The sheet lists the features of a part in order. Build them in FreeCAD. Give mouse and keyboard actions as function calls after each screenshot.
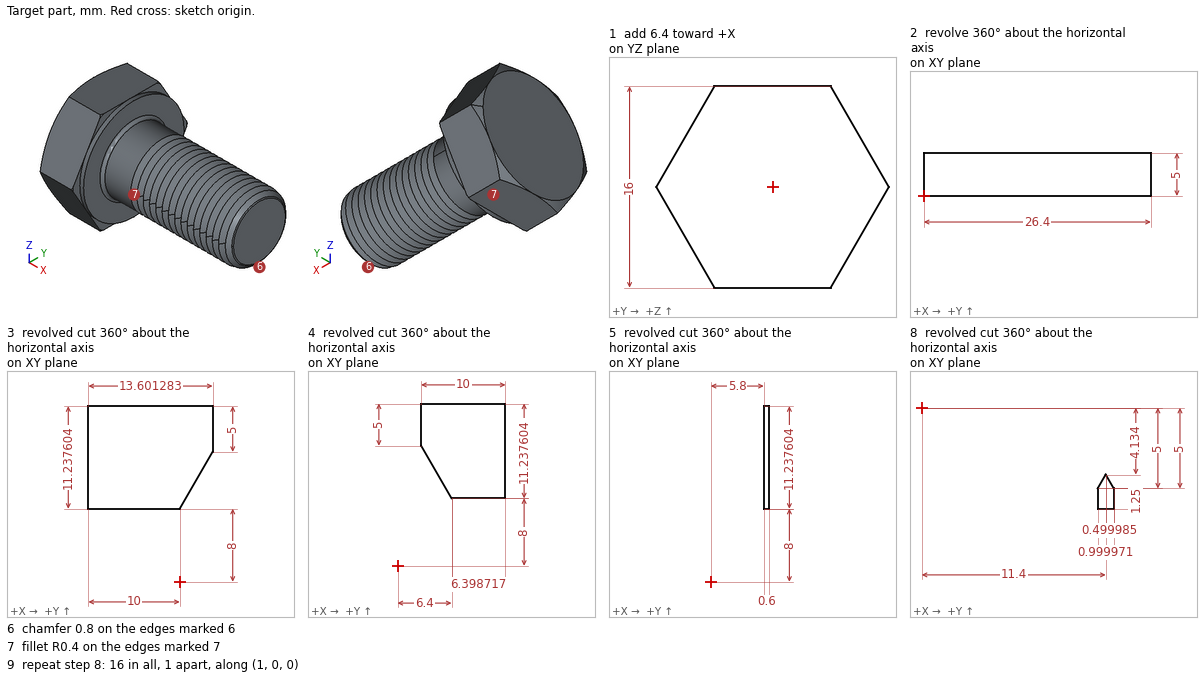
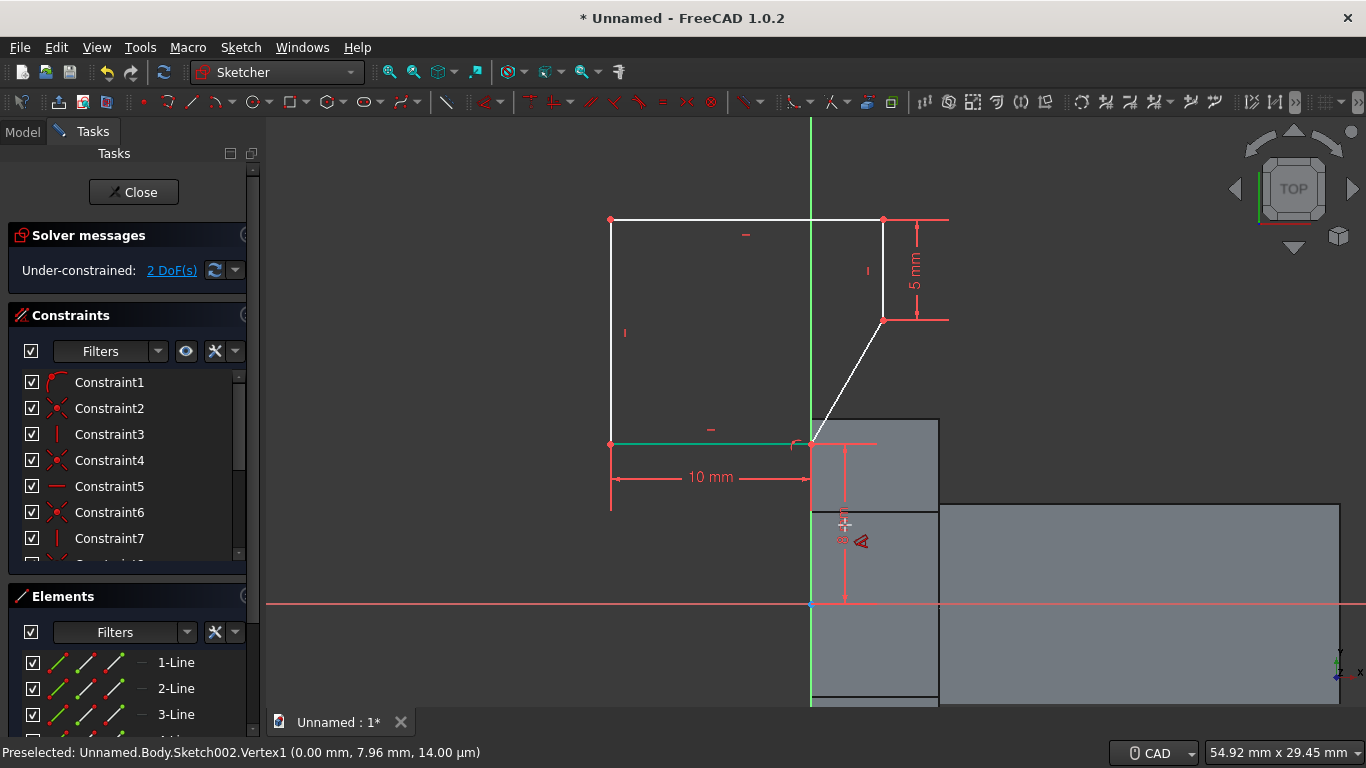
scroll(801, 220, up, 2)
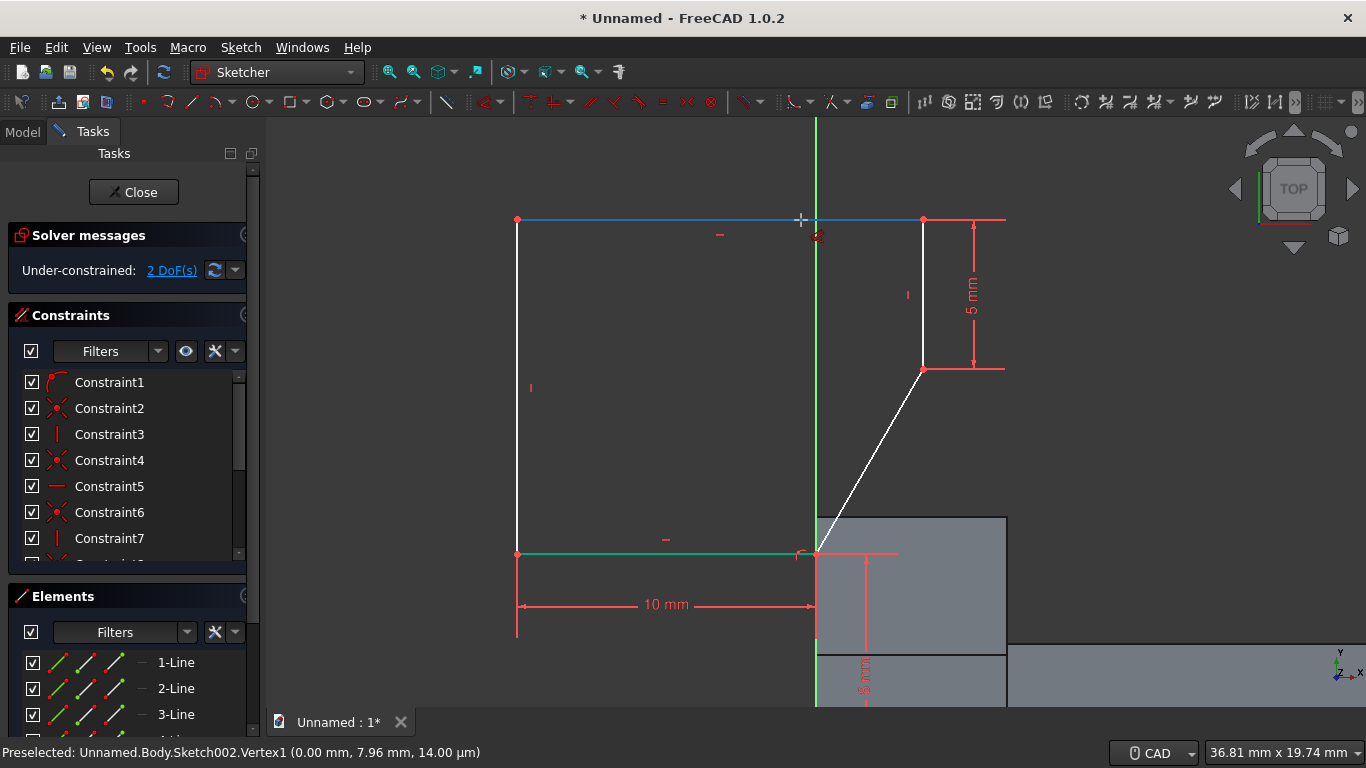
click(801, 220)
click(720, 186)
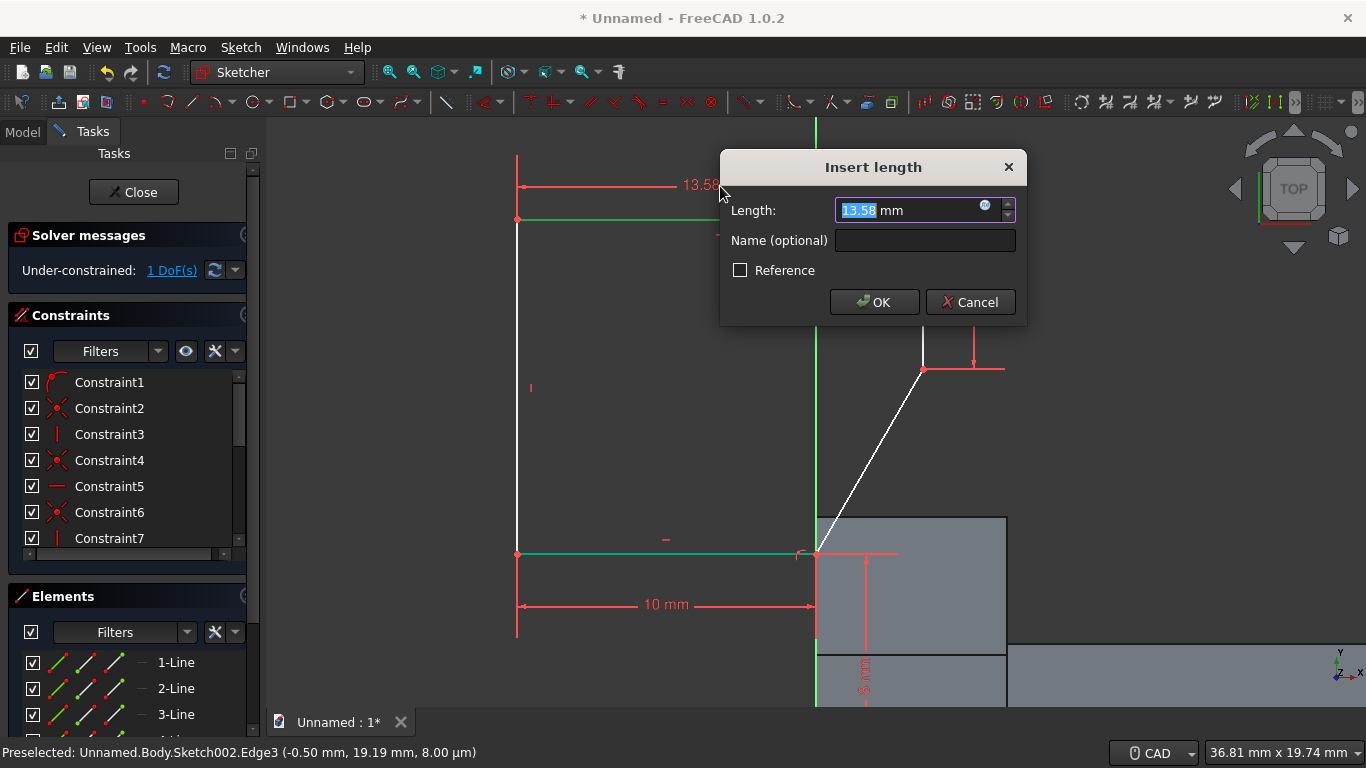
text(13.601283)
key(Return)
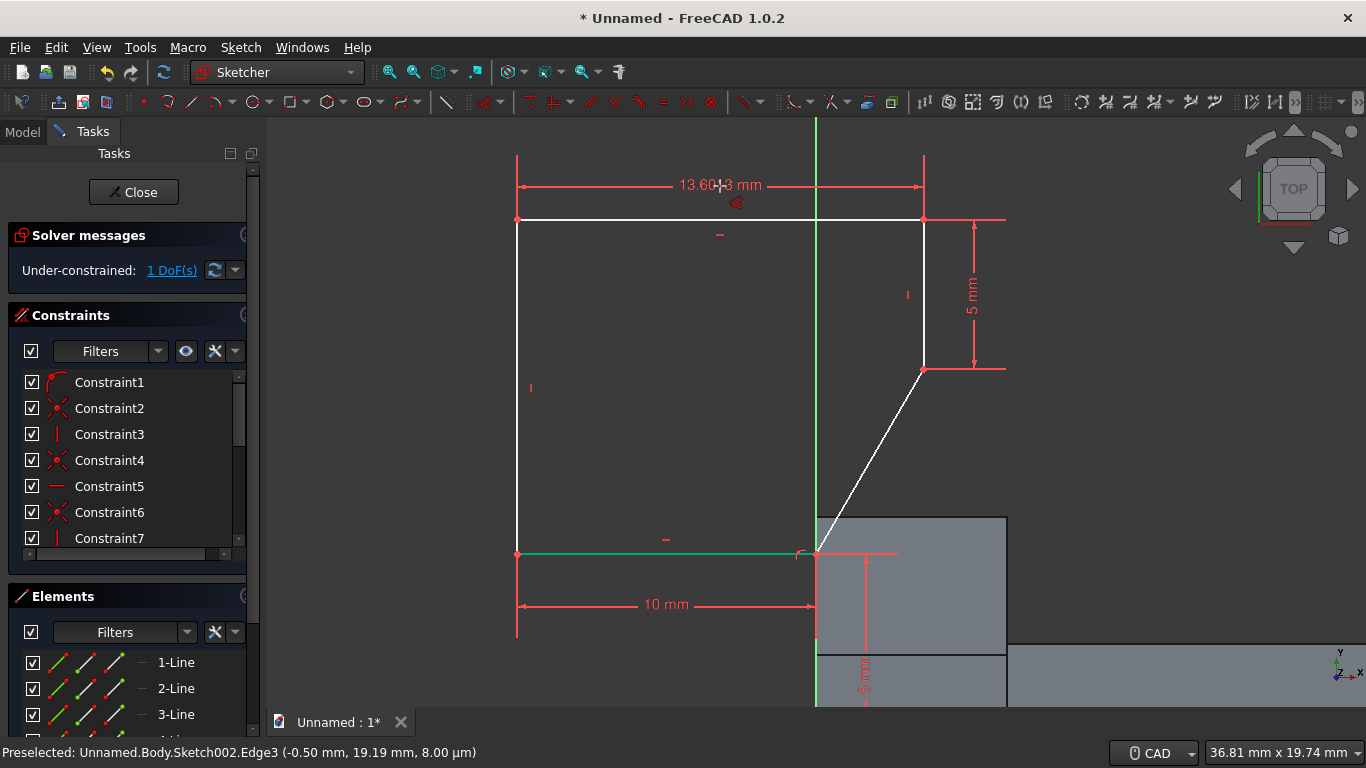
click(517, 320)
click(483, 387)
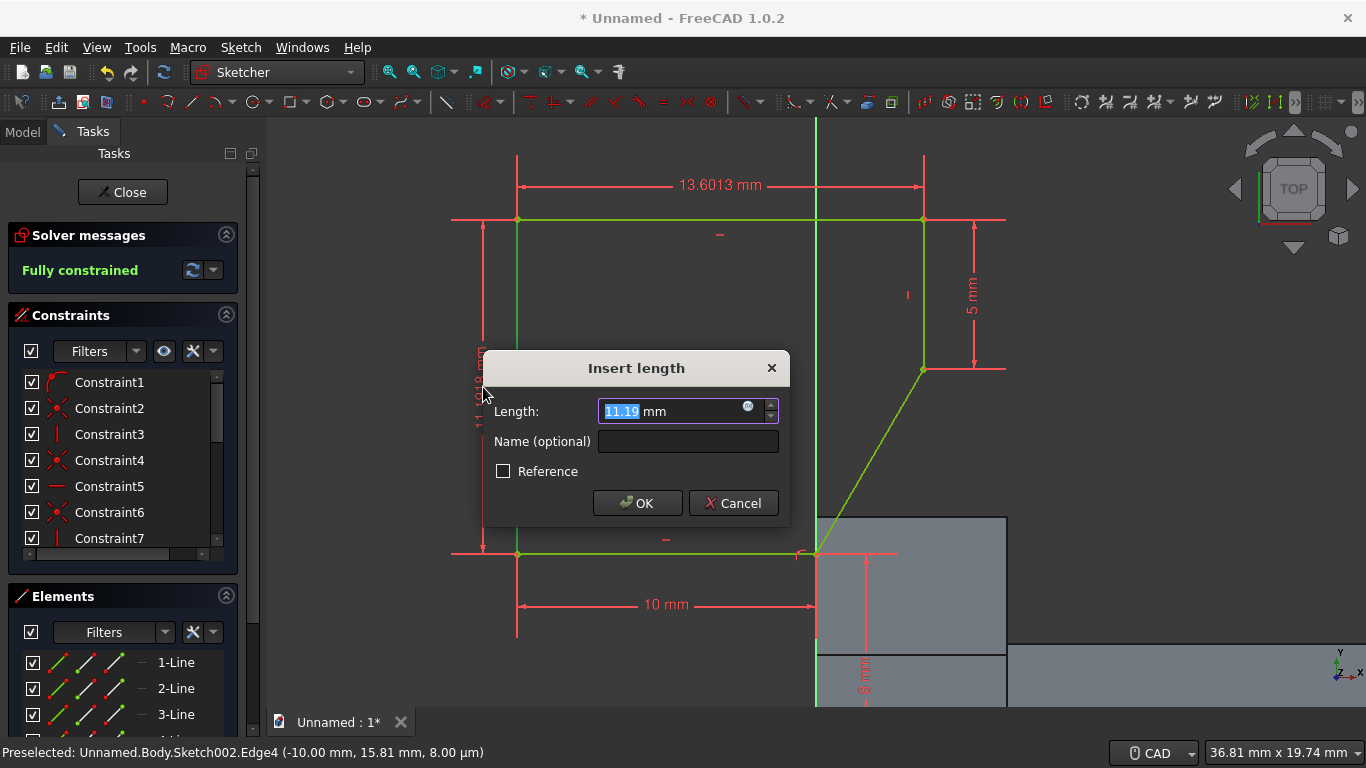
text(11.237604)
key(Return)
key(Escape)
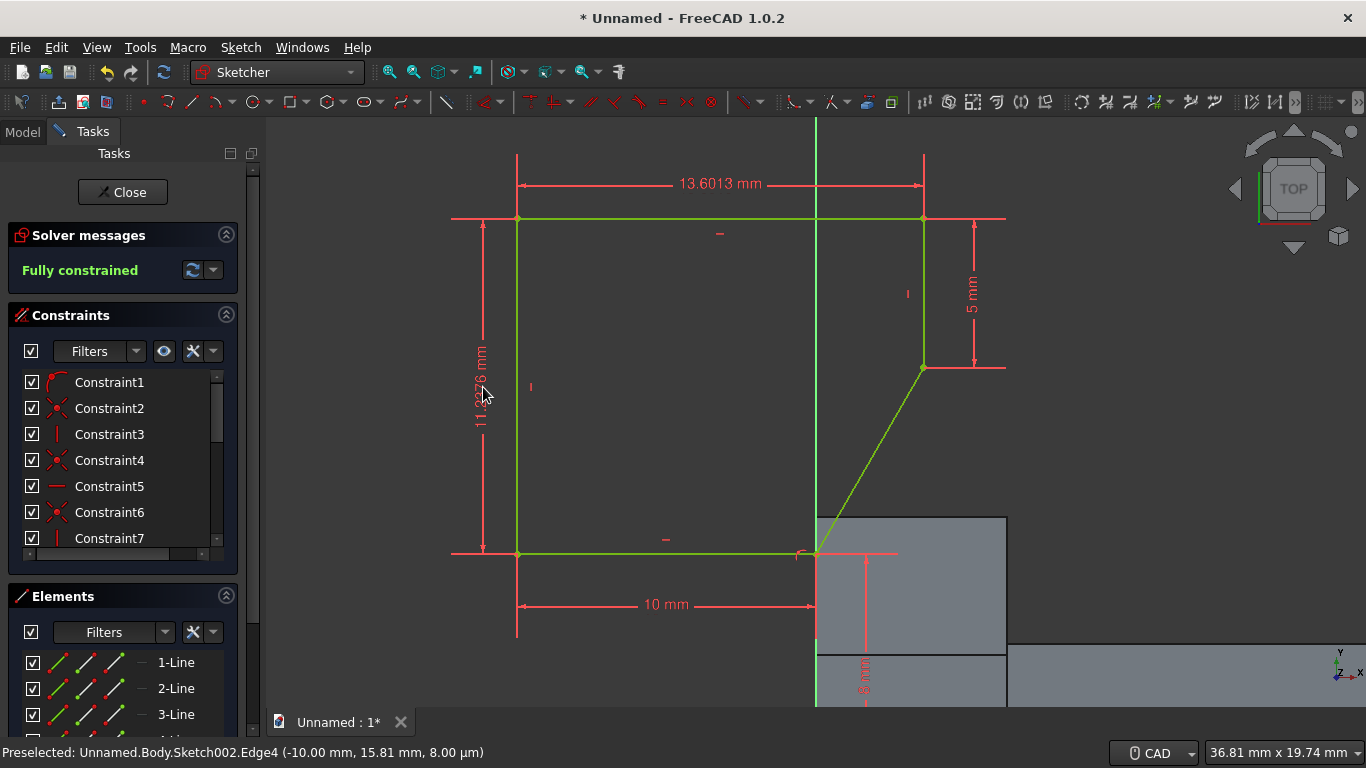
click(123, 192)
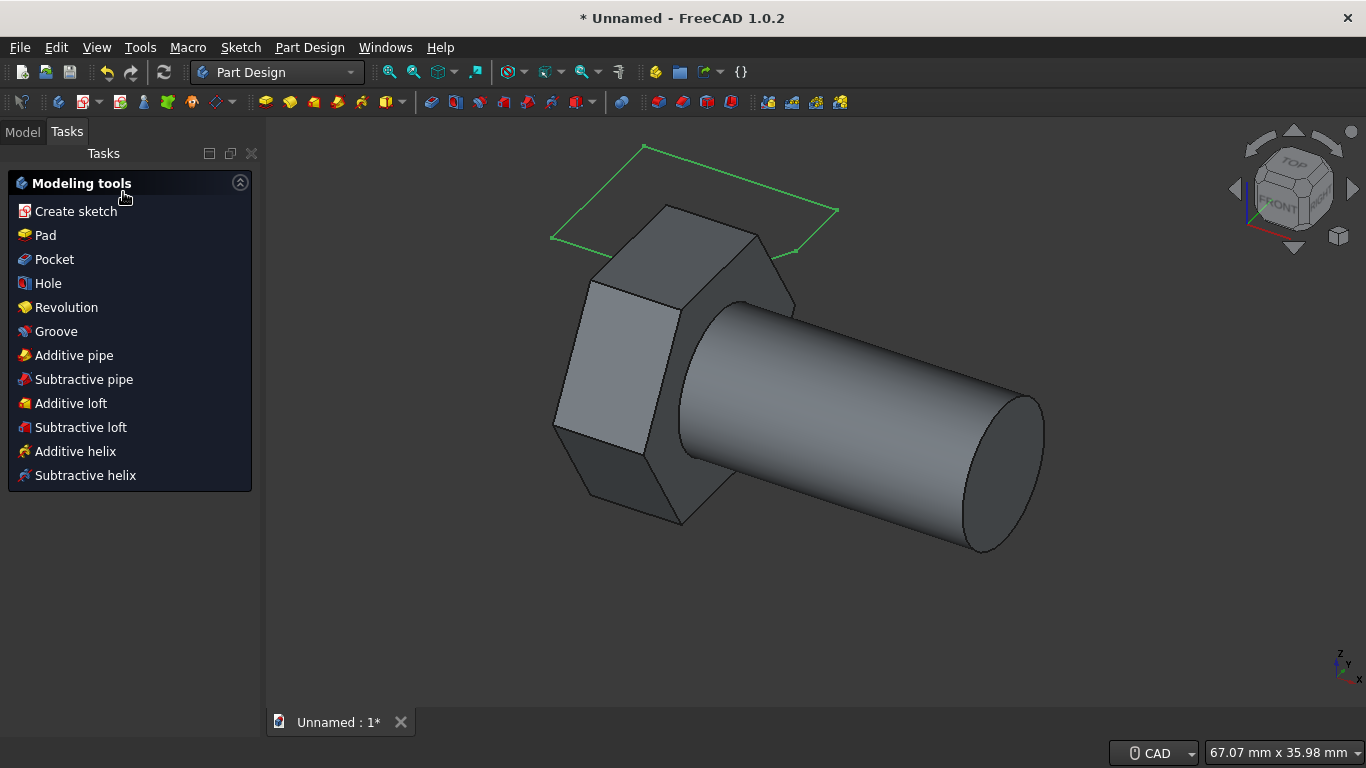
click(480, 102)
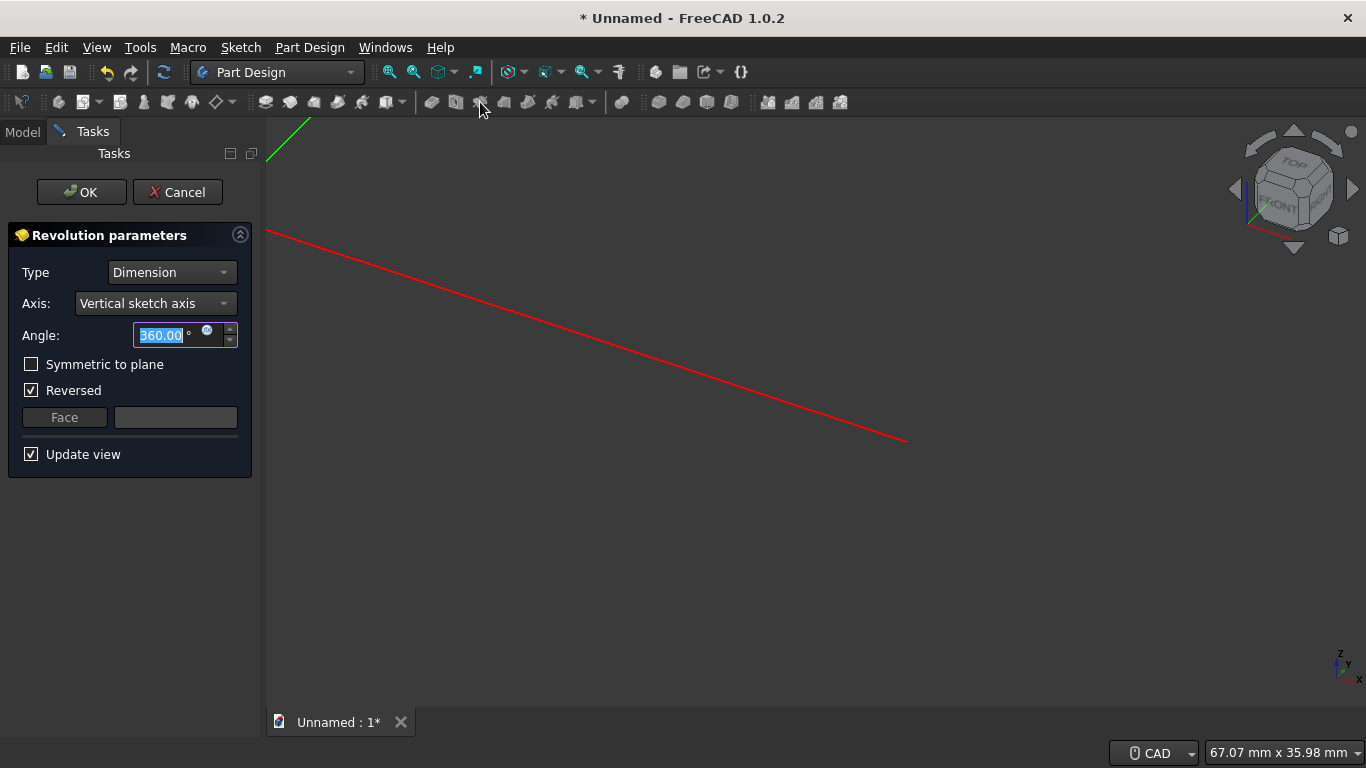
click(156, 304)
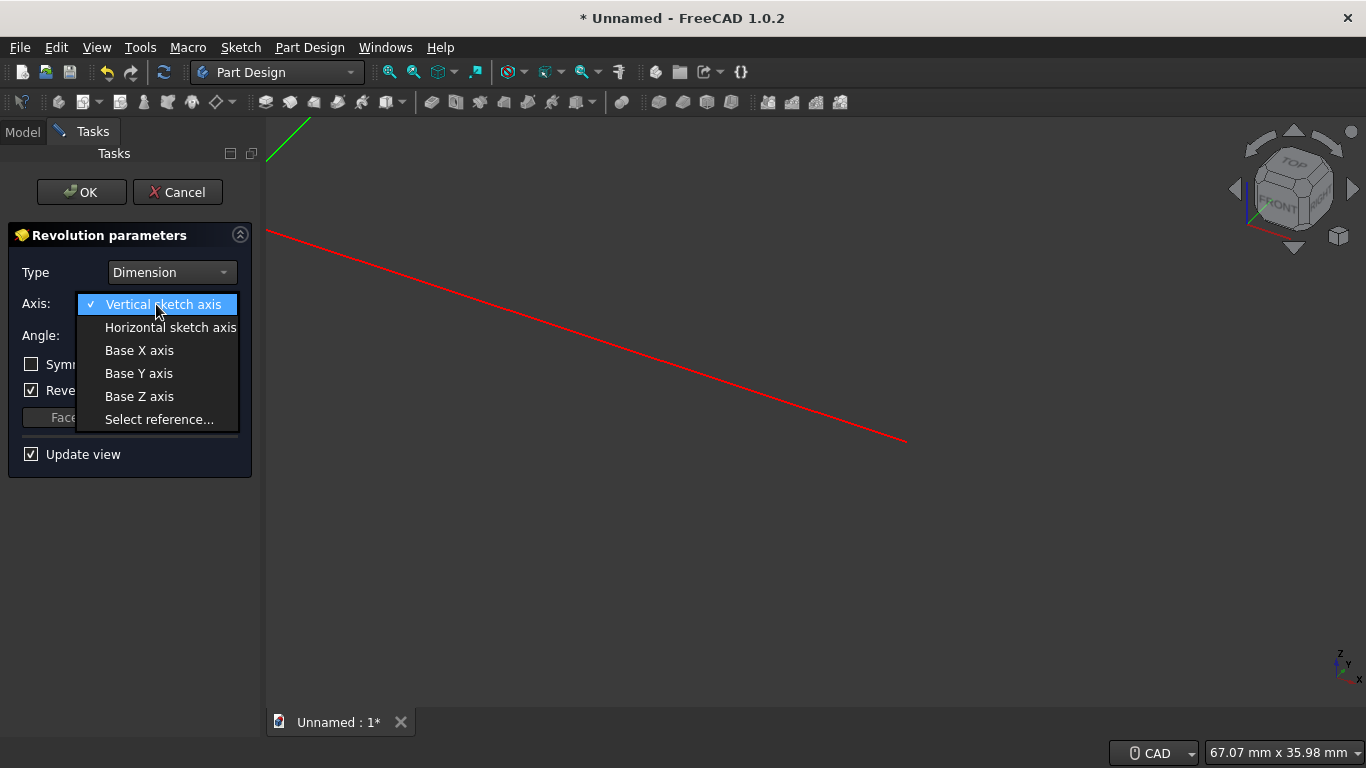
click(156, 328)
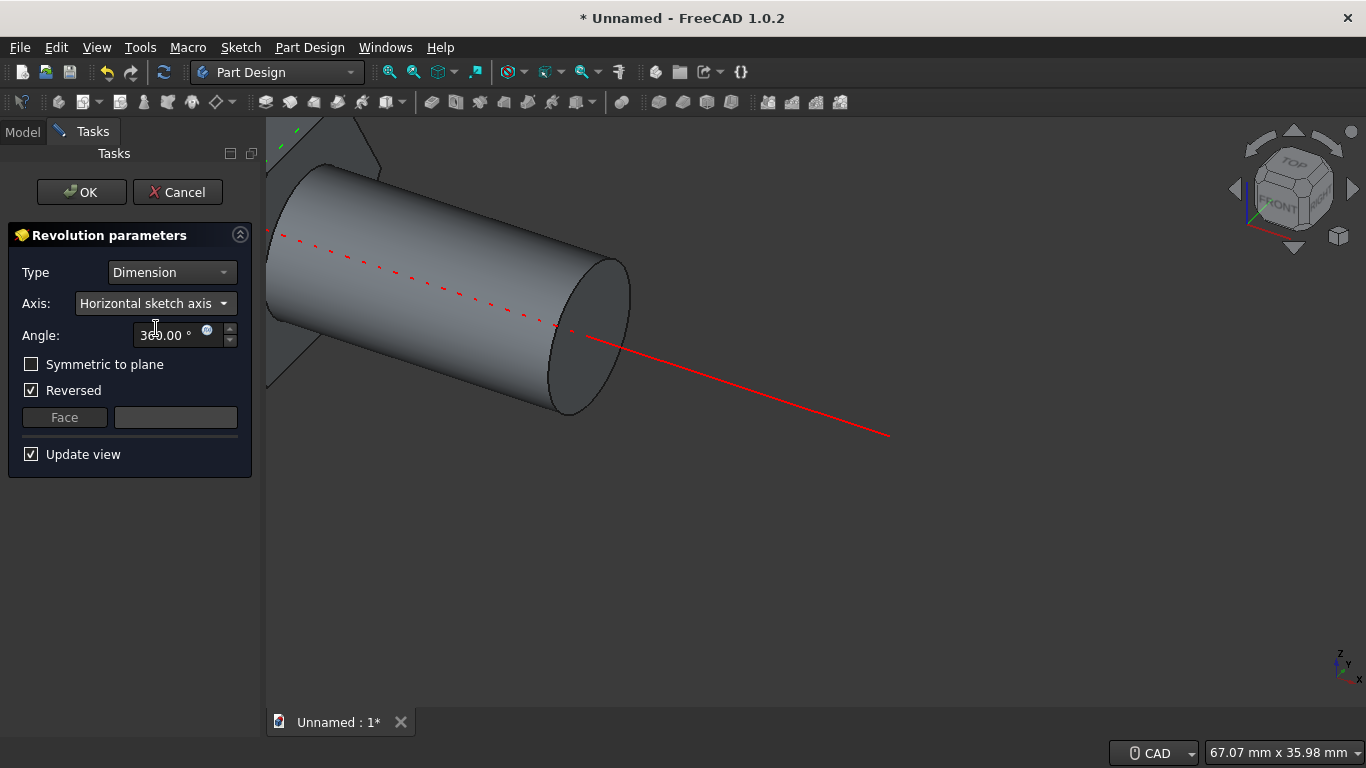
click(82, 192)